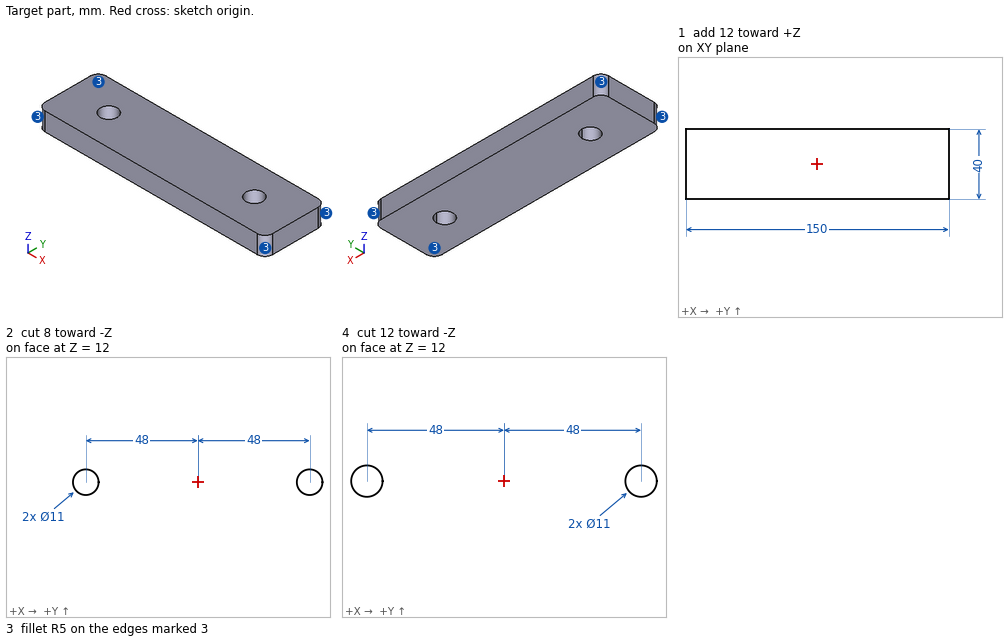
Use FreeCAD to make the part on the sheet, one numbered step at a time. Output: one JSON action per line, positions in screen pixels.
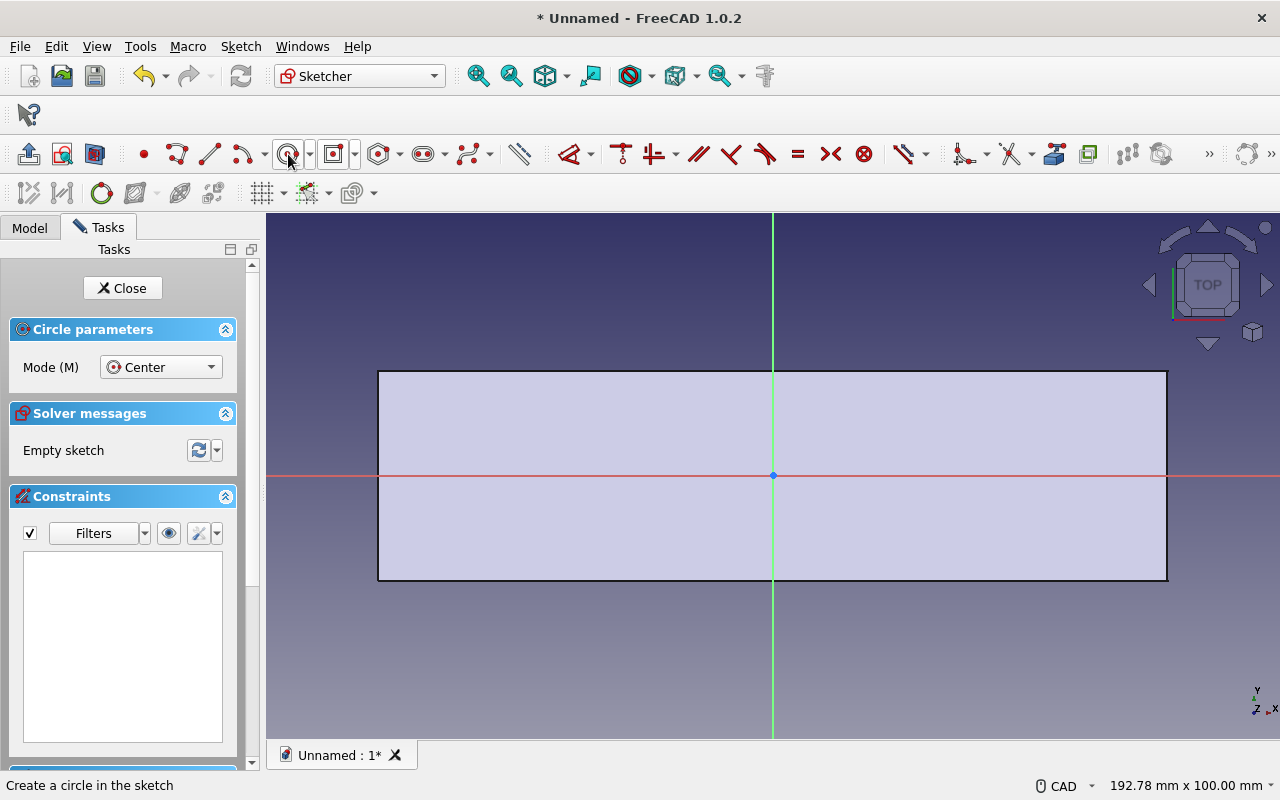
{"action": "left_click", "coordinate": [521, 476]}
{"action": "left_click", "coordinate": [541, 456]}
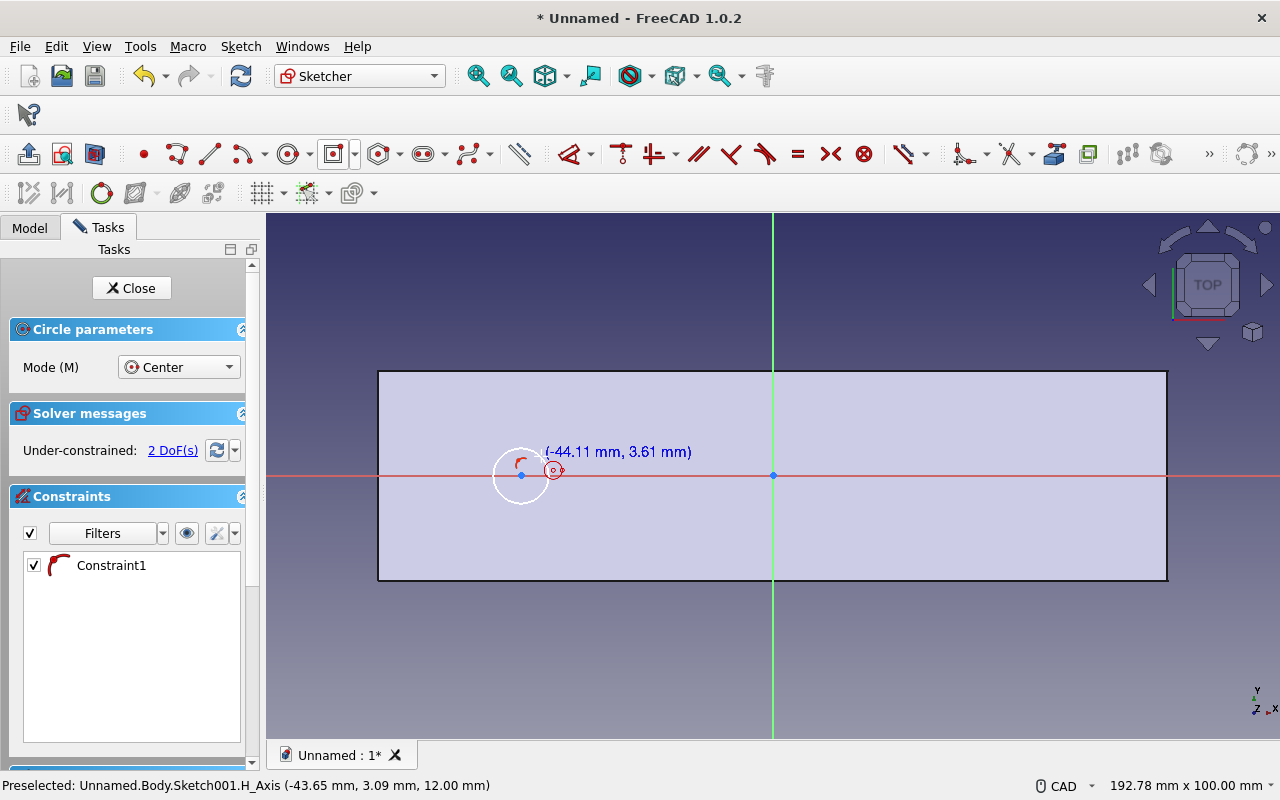
{"action": "left_click", "coordinate": [1025, 476]}
{"action": "left_click", "coordinate": [1046, 456]}
{"action": "key", "text": "Escape"}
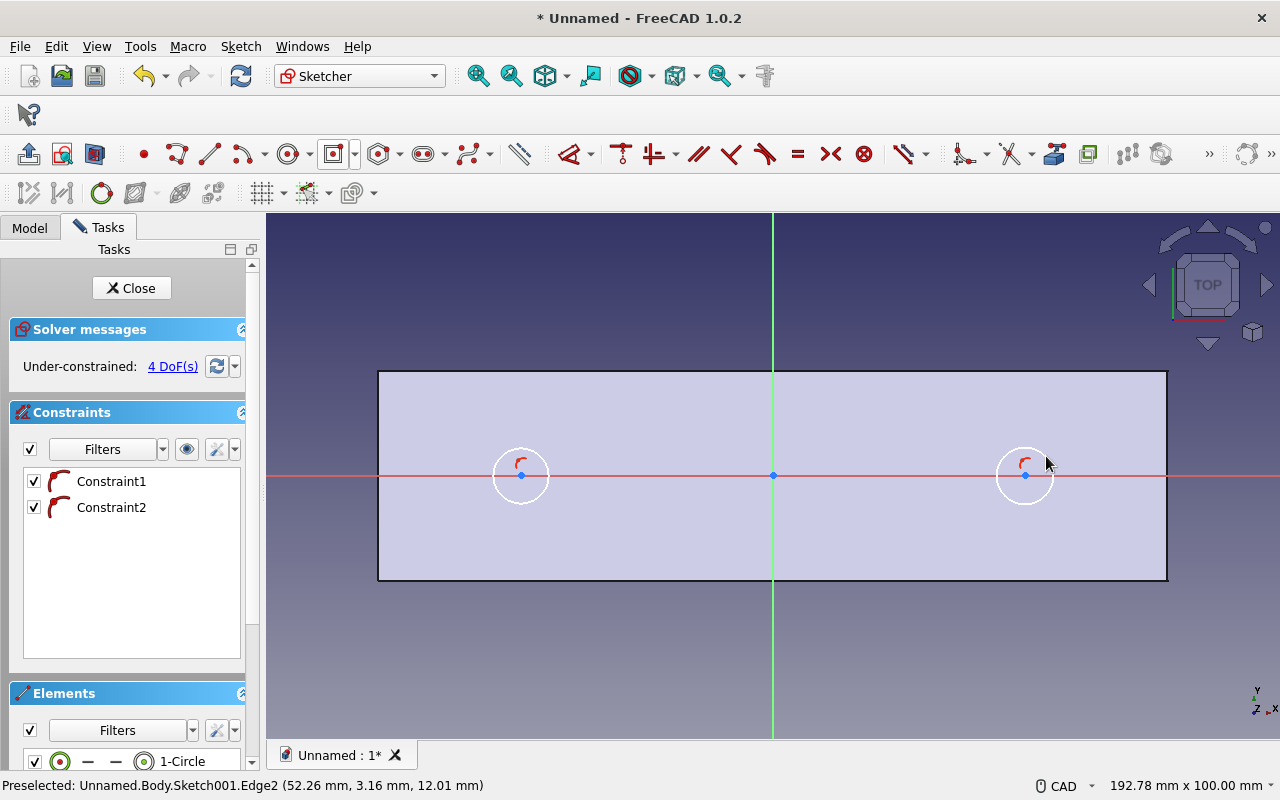
{"action": "left_click", "coordinate": [540, 456]}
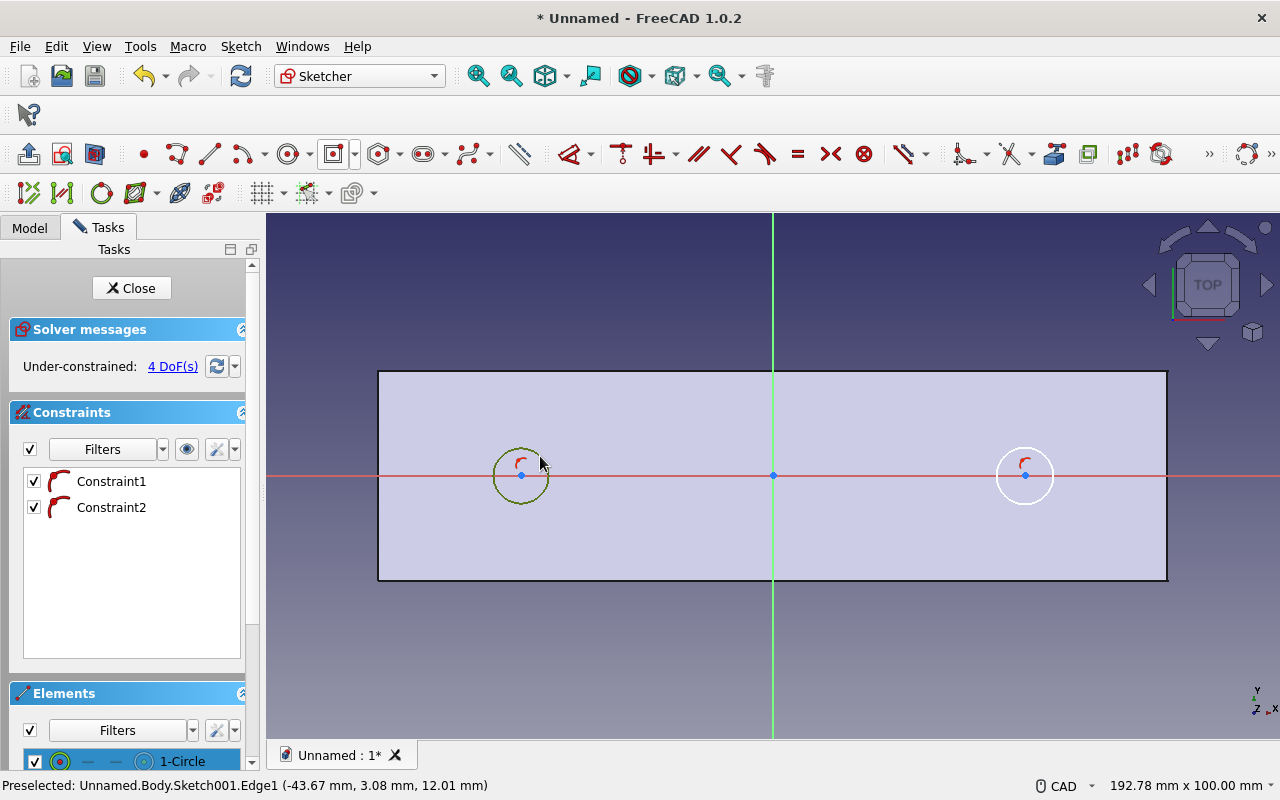
{"action": "left_click", "coordinate": [1045, 456]}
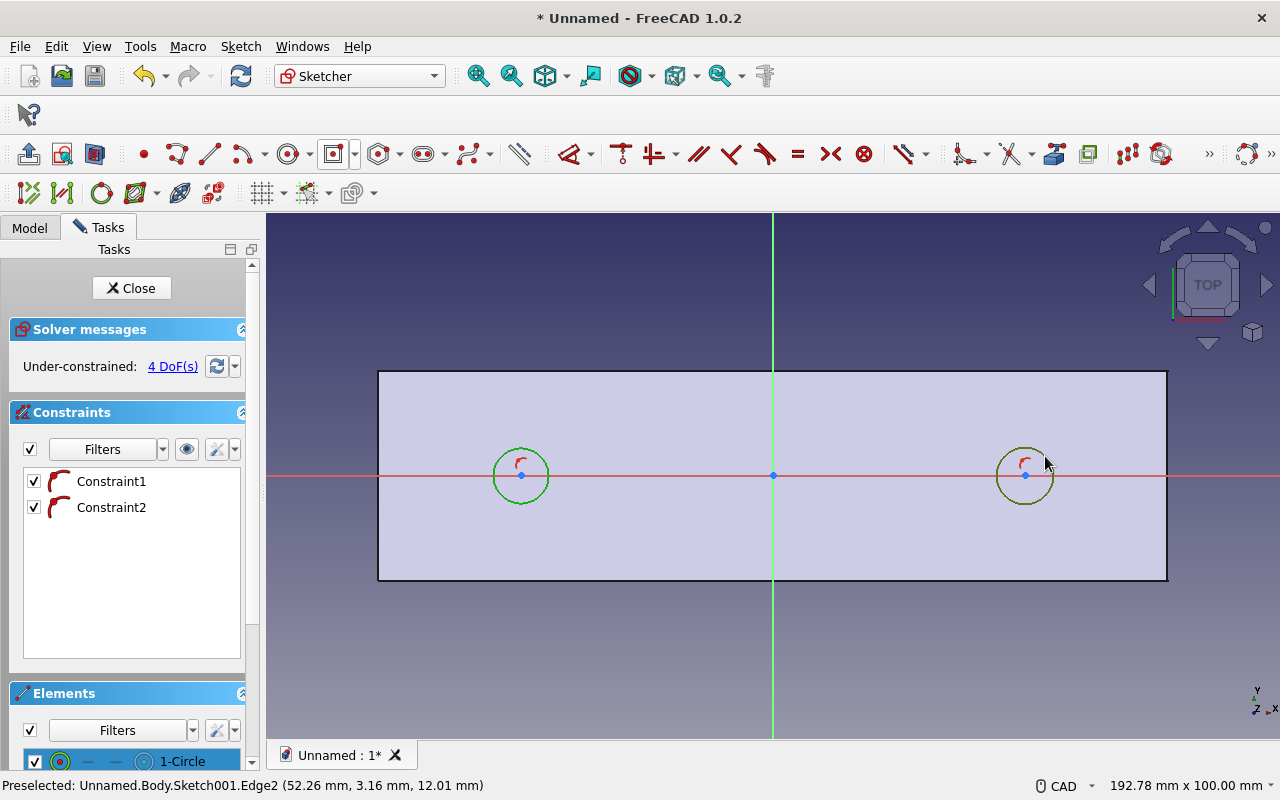
{"action": "left_click", "coordinate": [798, 154]}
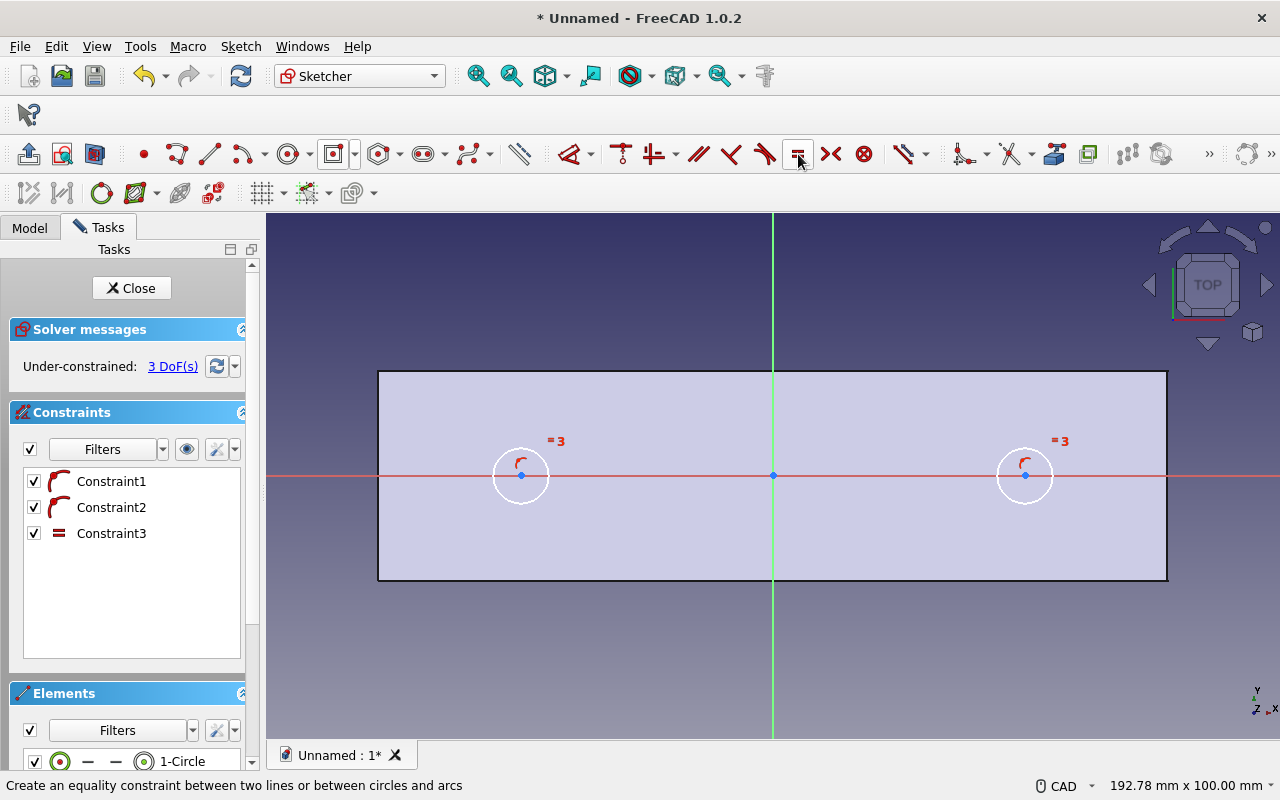
{"action": "left_click", "coordinate": [568, 154]}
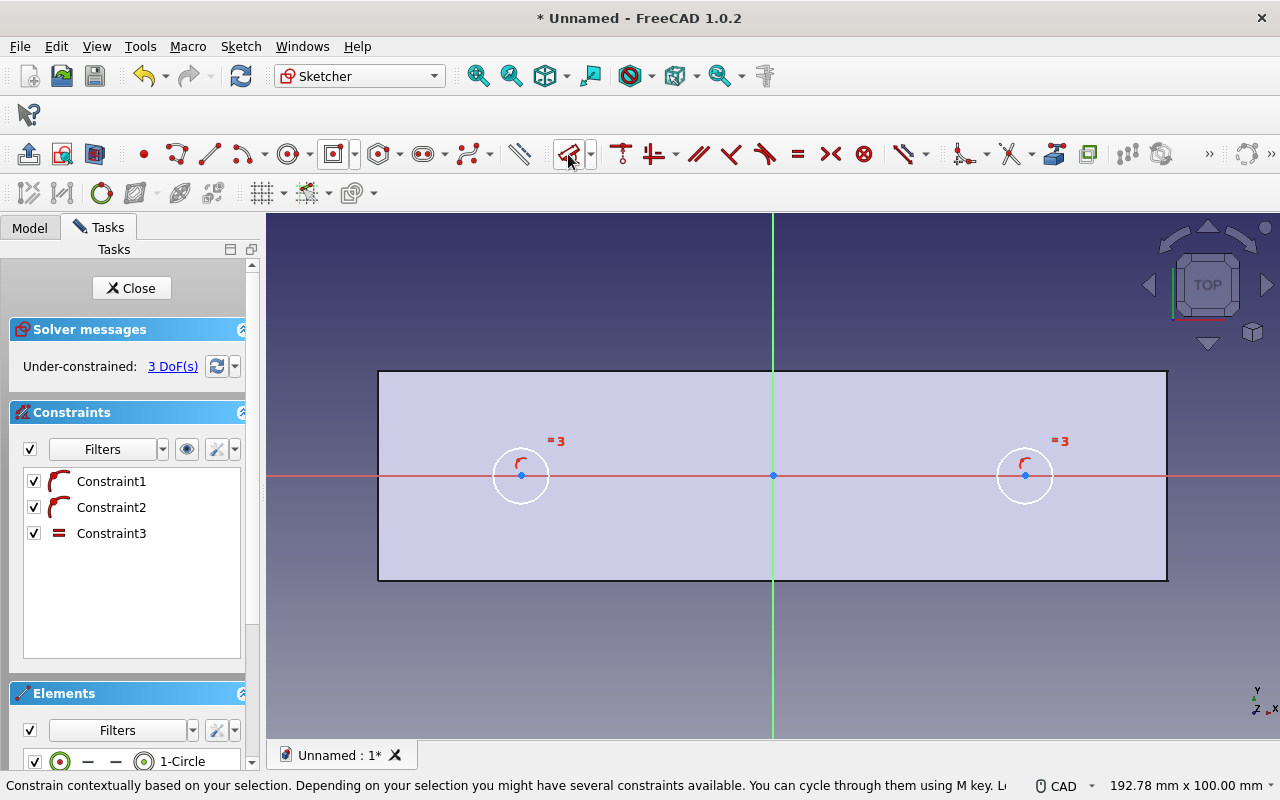
{"action": "left_click", "coordinate": [540, 456]}
{"action": "left_click", "coordinate": [562, 433]}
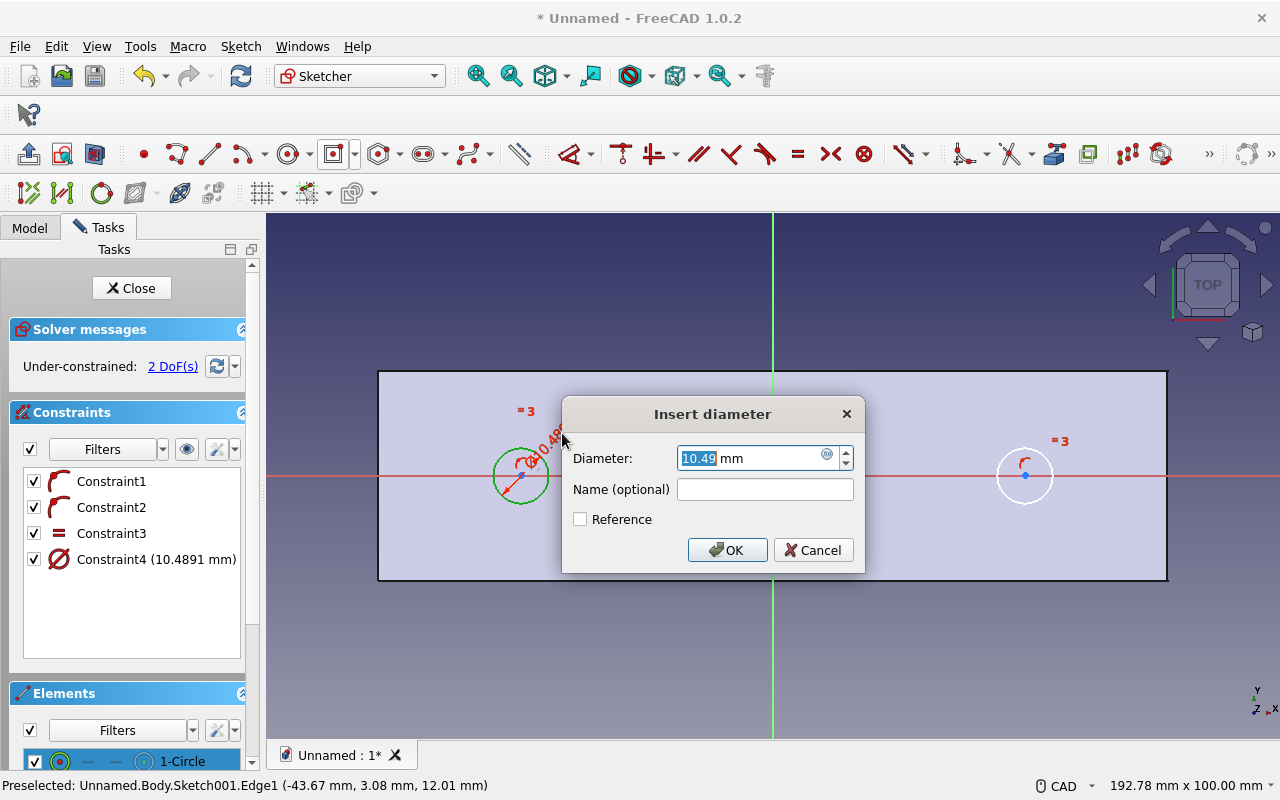
{"action": "type", "text": "11"}
{"action": "key", "text": "Return"}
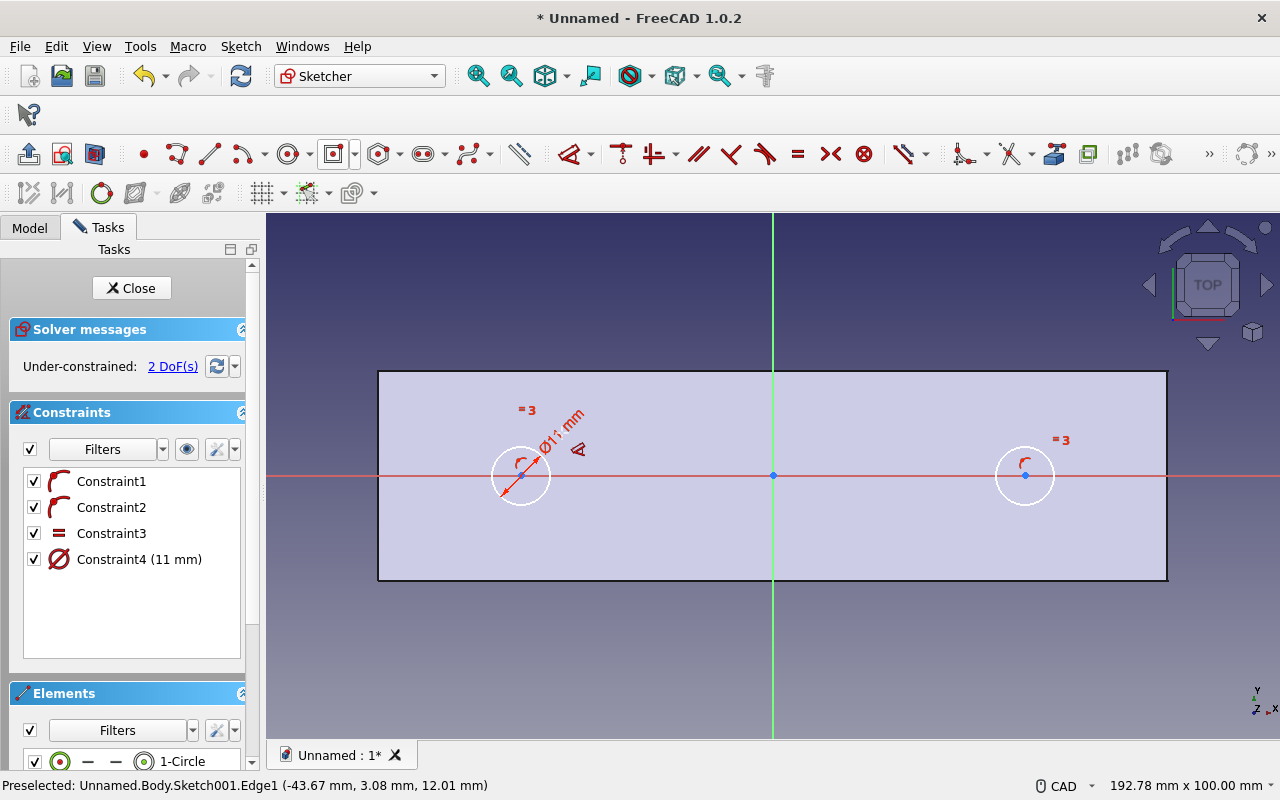
{"action": "left_click", "coordinate": [521, 476]}
{"action": "left_click", "coordinate": [647, 510]}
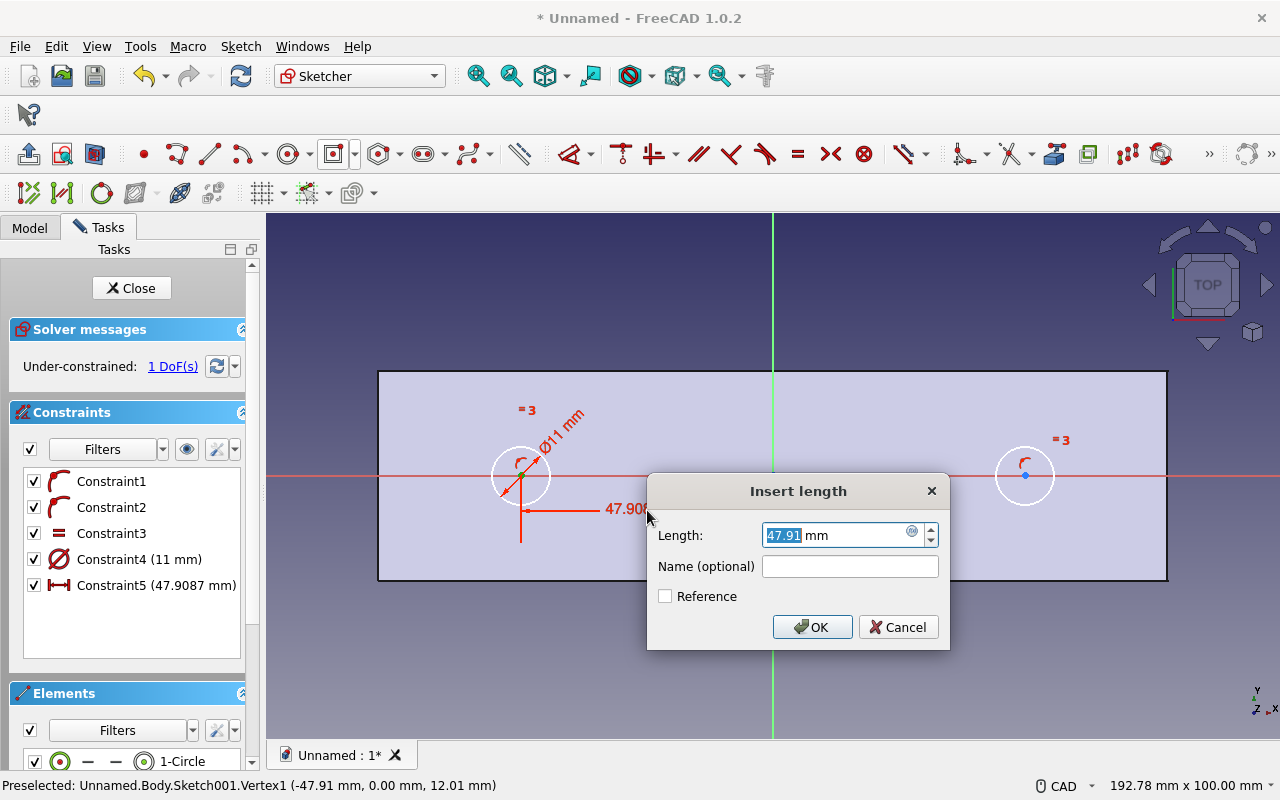
{"action": "type", "text": "48"}
{"action": "key", "text": "Return"}